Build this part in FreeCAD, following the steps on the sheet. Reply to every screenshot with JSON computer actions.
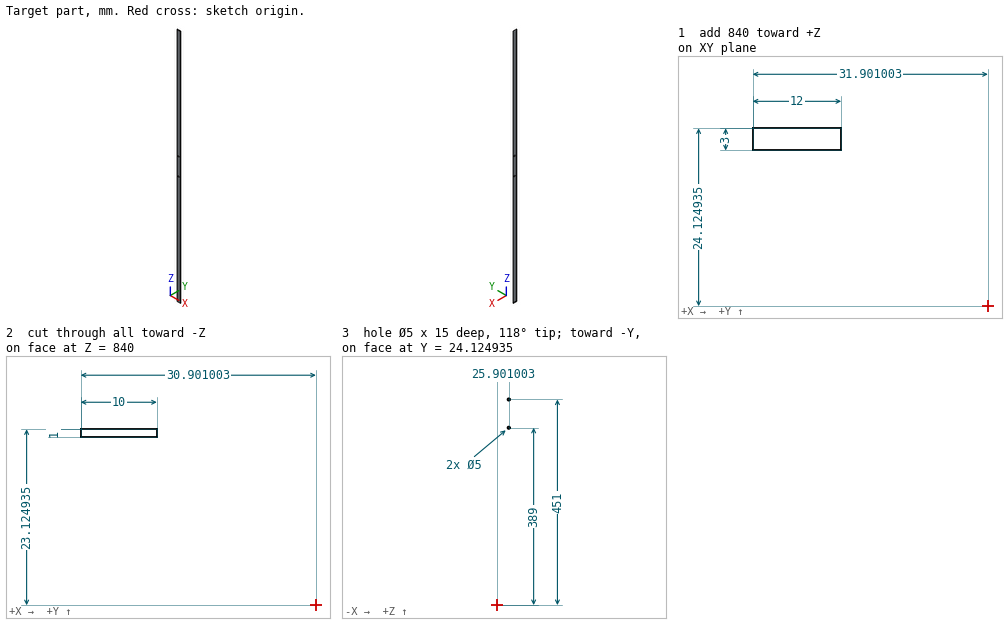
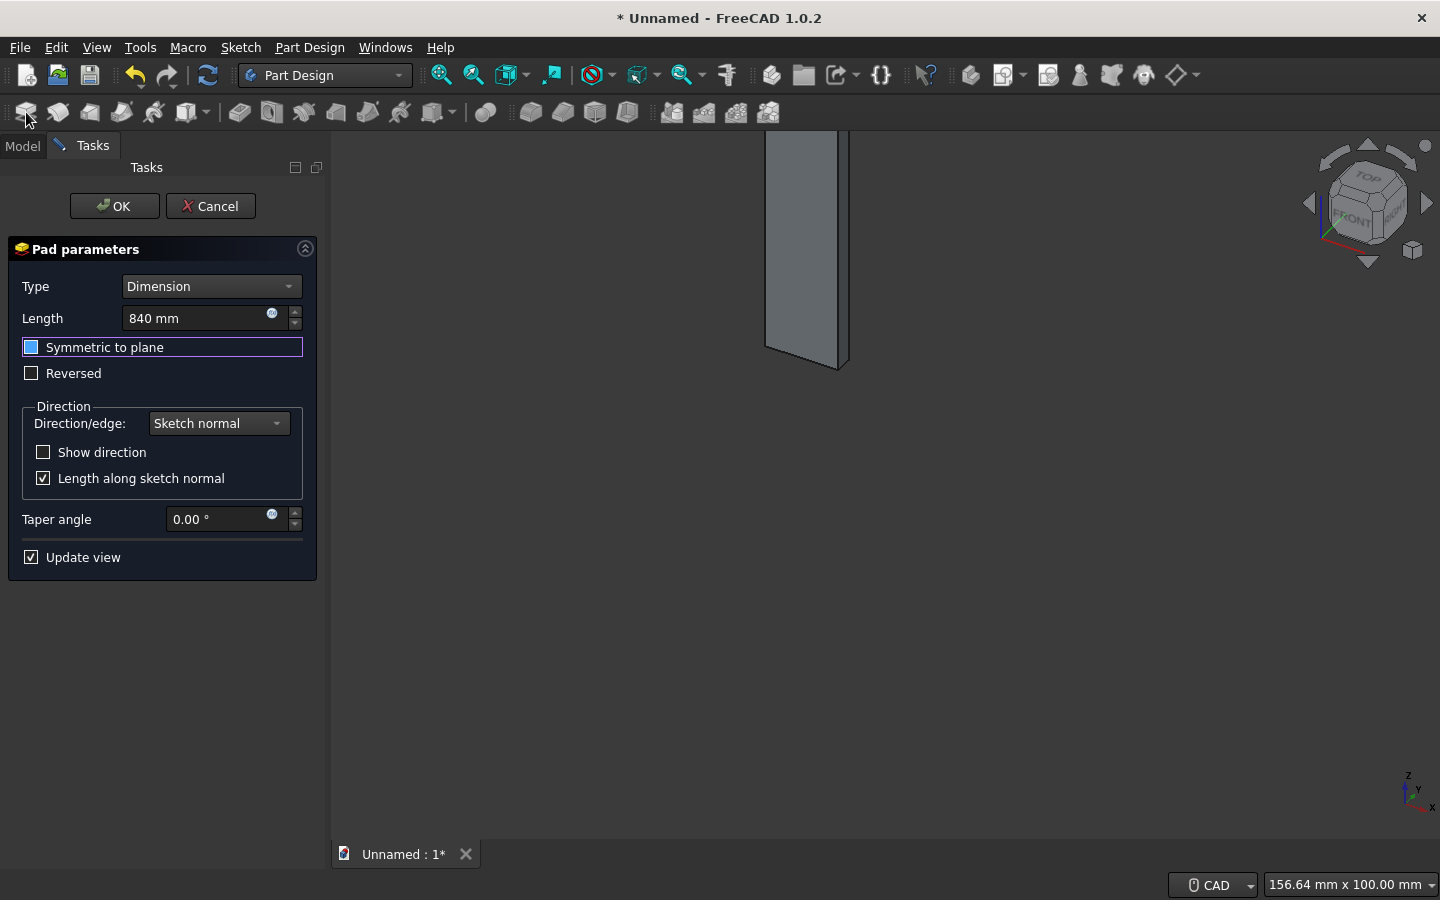
{"action": "left_click", "coordinate": [115, 206]}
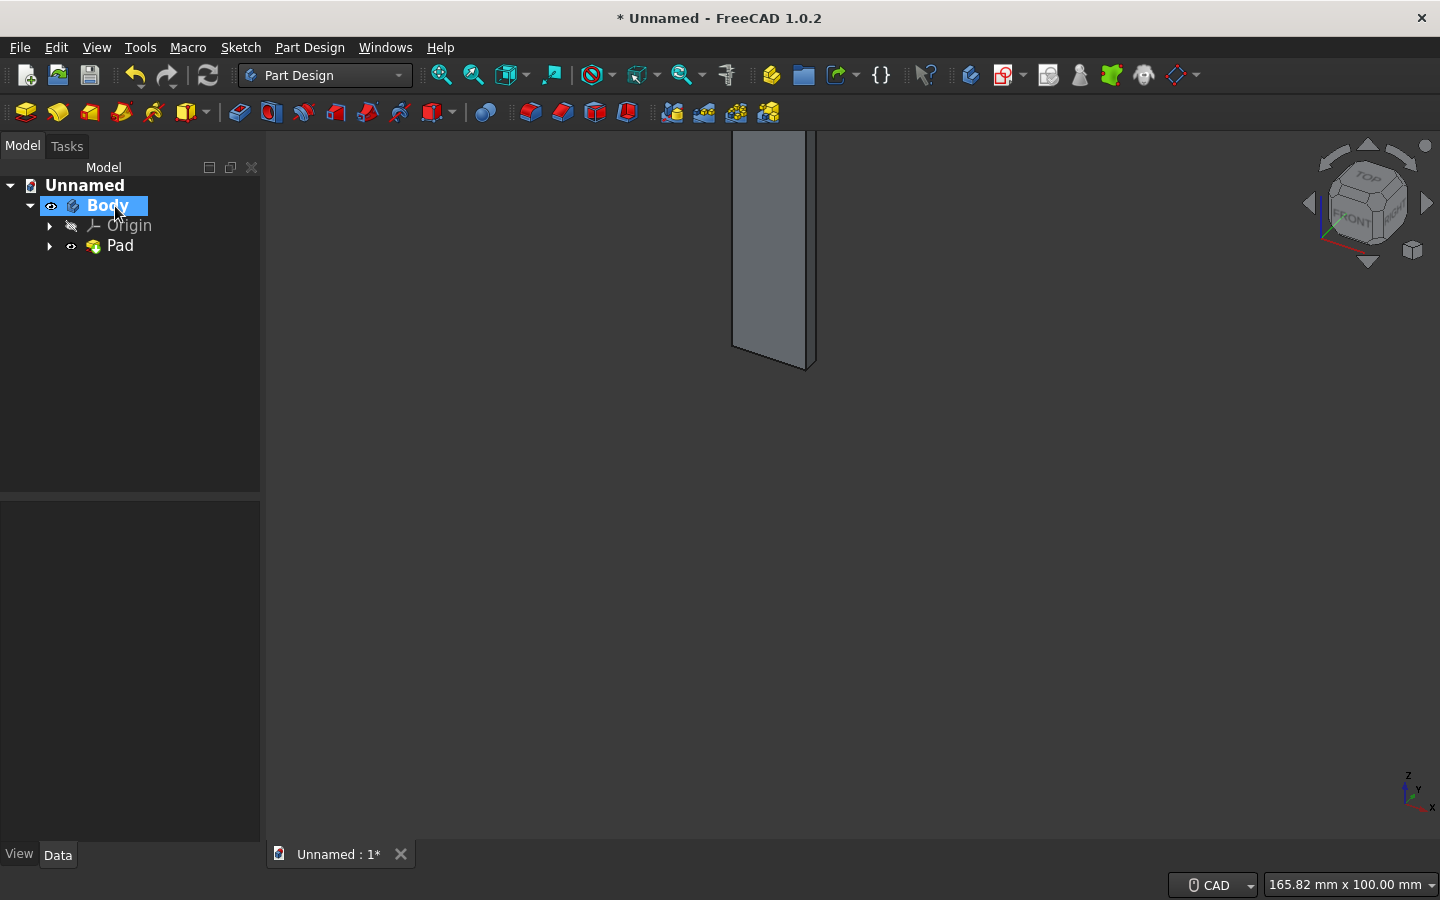
{"action": "left_click", "coordinate": [442, 76]}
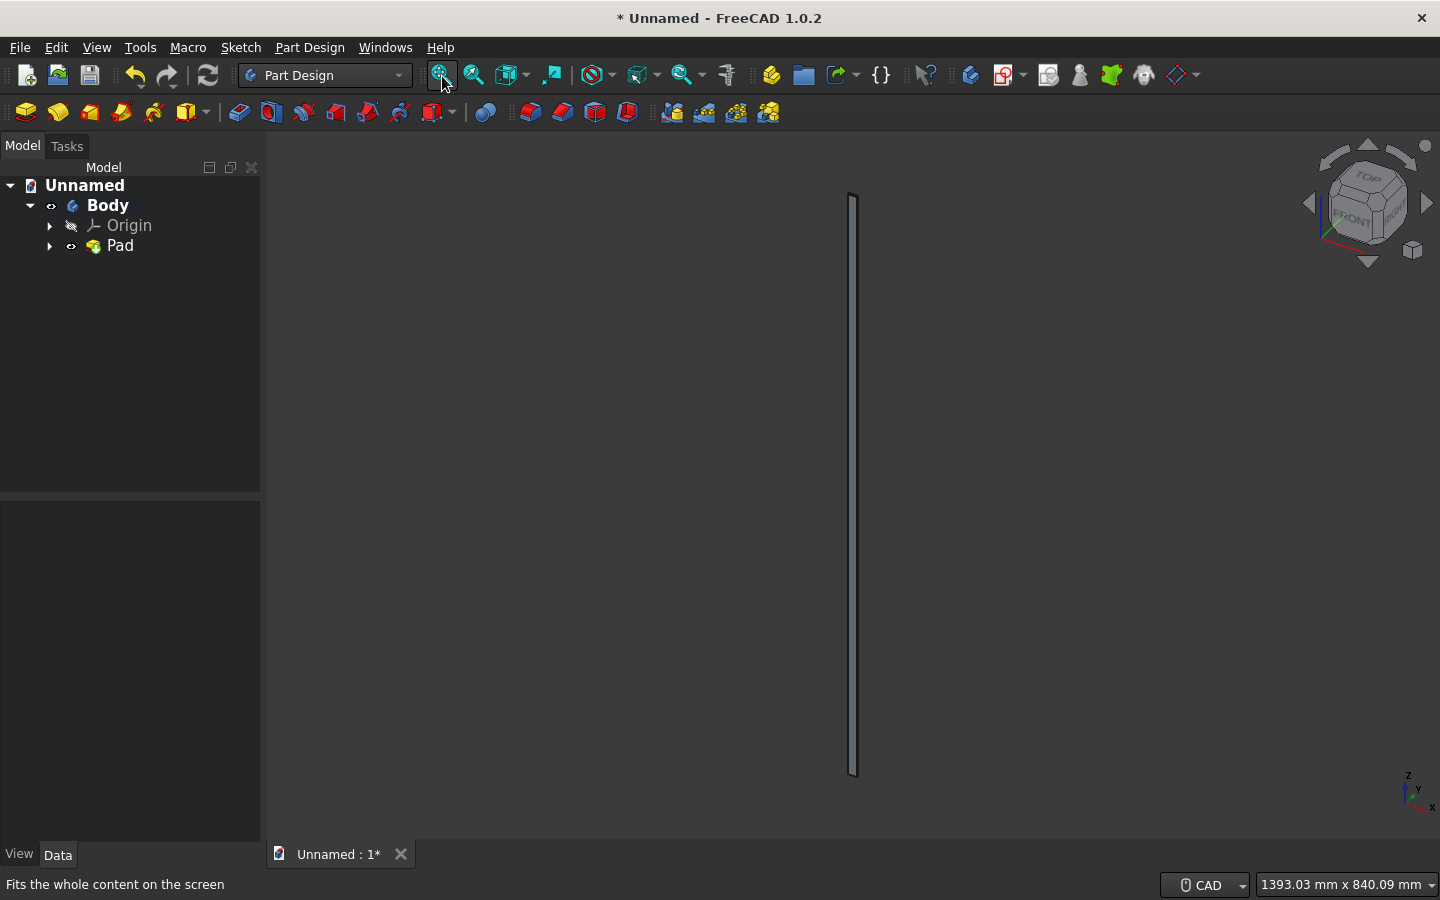
{"action": "scroll", "coordinate": [856, 195], "scroll_direction": "up", "scroll_amount": 12}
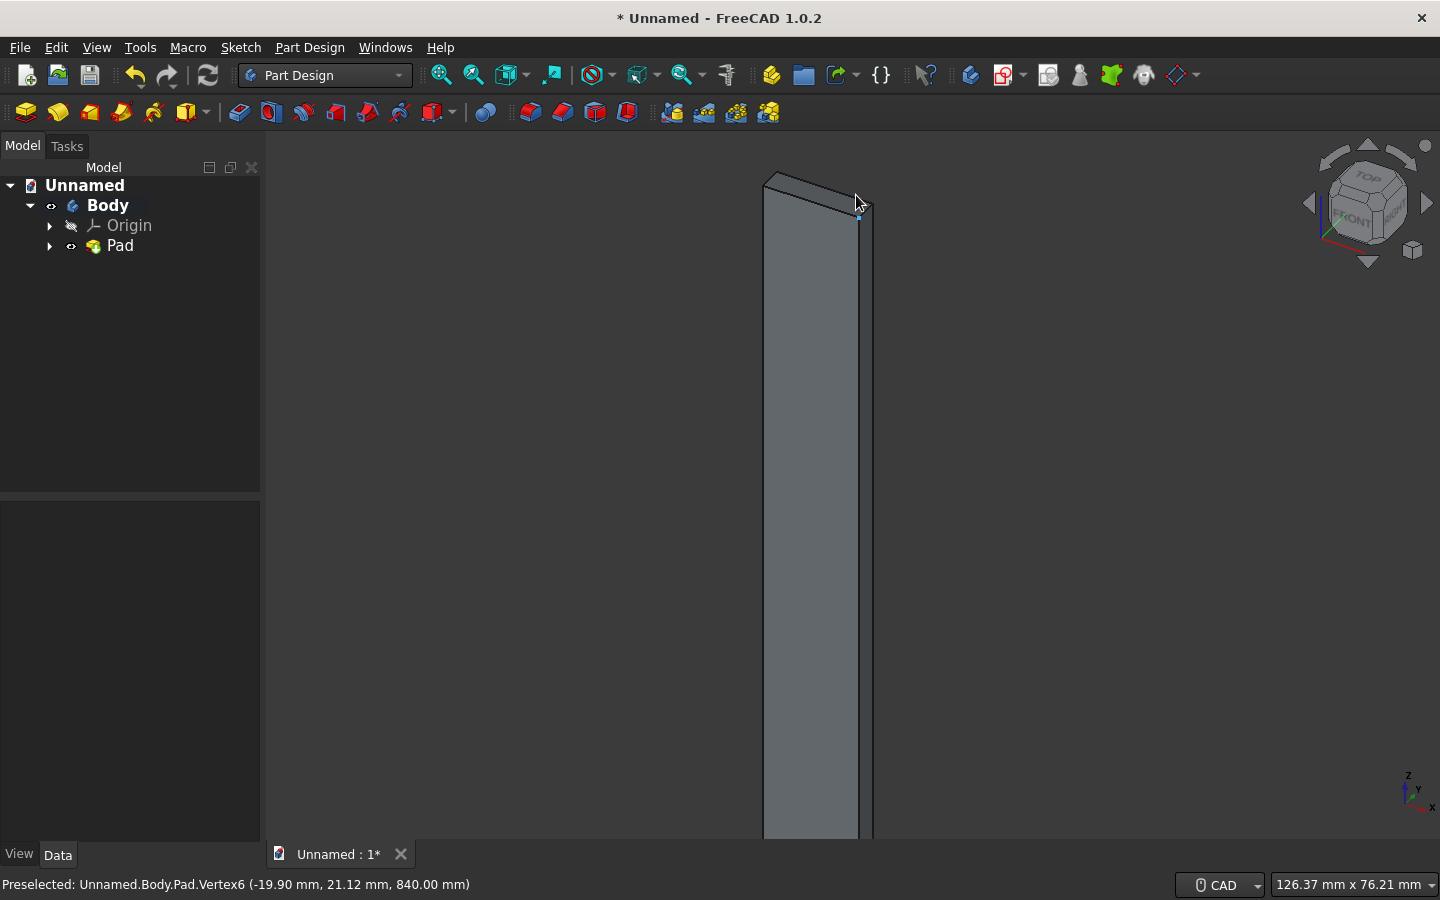
{"action": "left_click", "coordinate": [832, 198]}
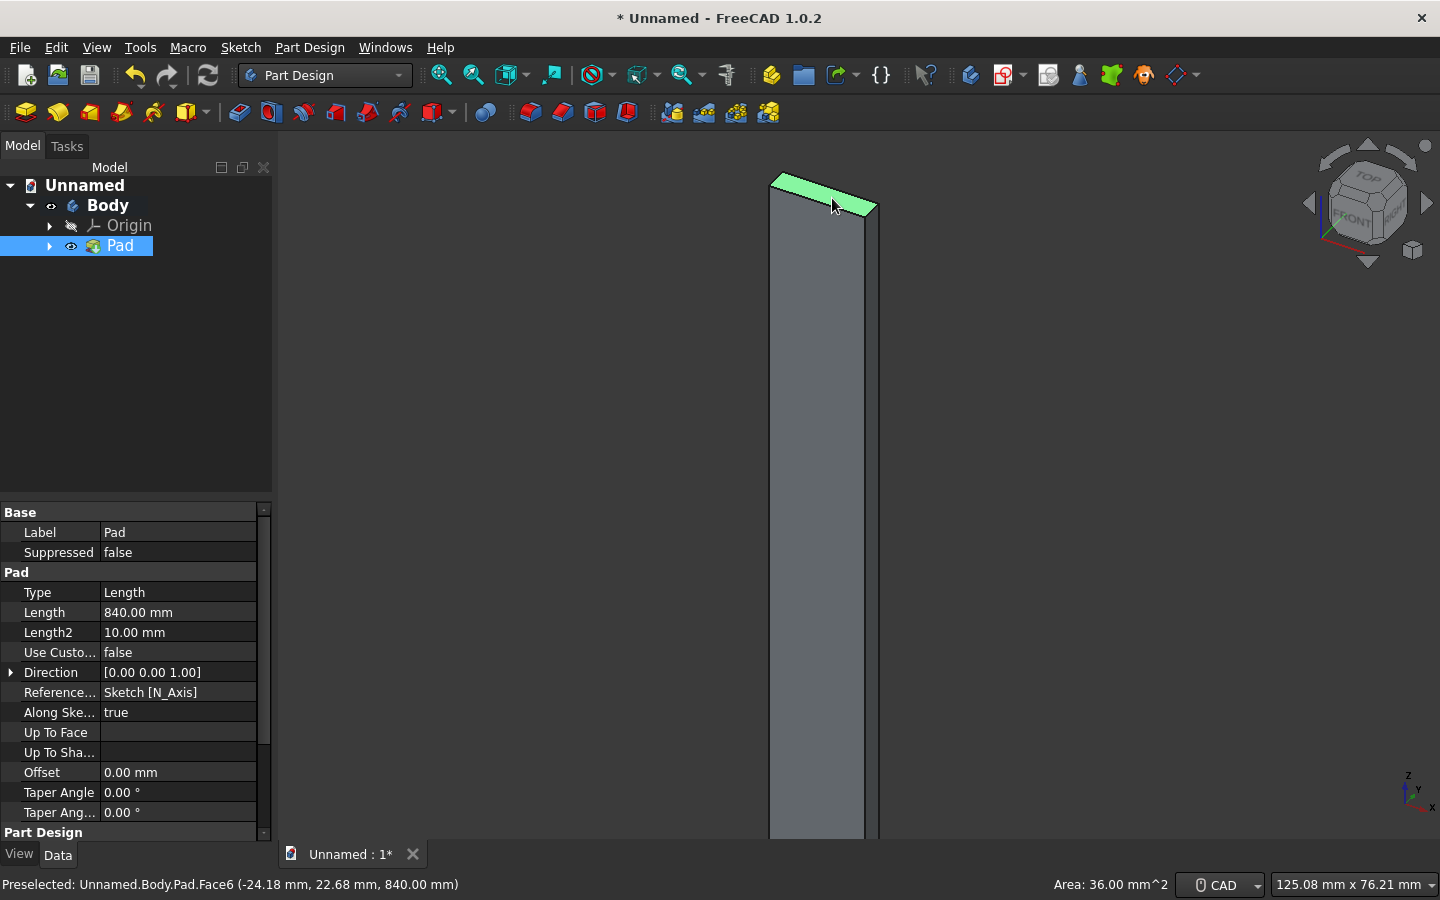
{"action": "left_click", "coordinate": [1004, 76]}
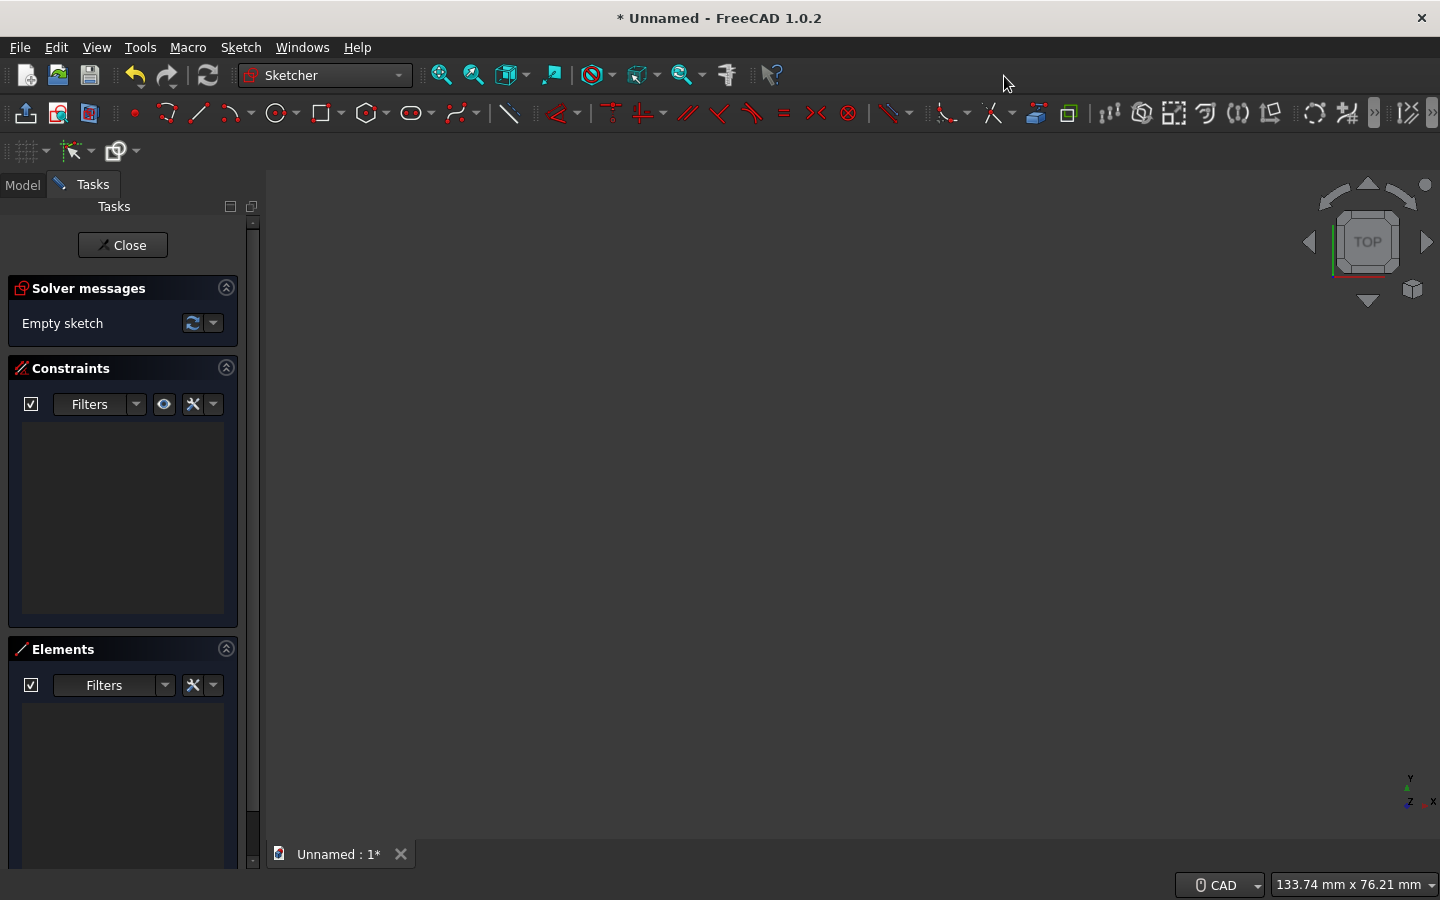
{"action": "scroll", "coordinate": [784, 504], "scroll_direction": "down", "scroll_amount": 5}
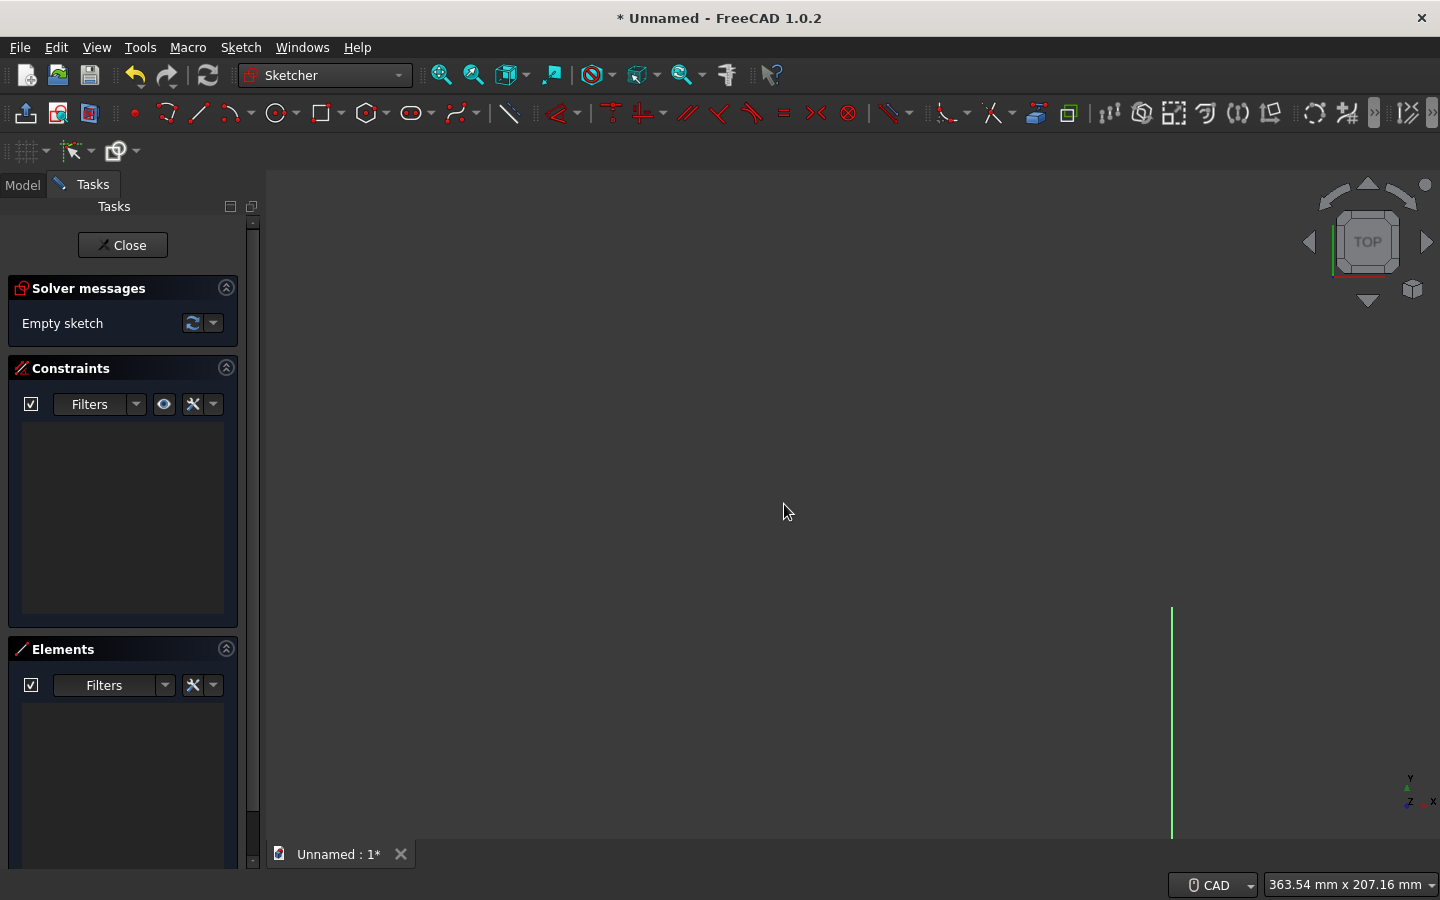
{"action": "scroll", "coordinate": [784, 504], "scroll_direction": "down", "scroll_amount": 5}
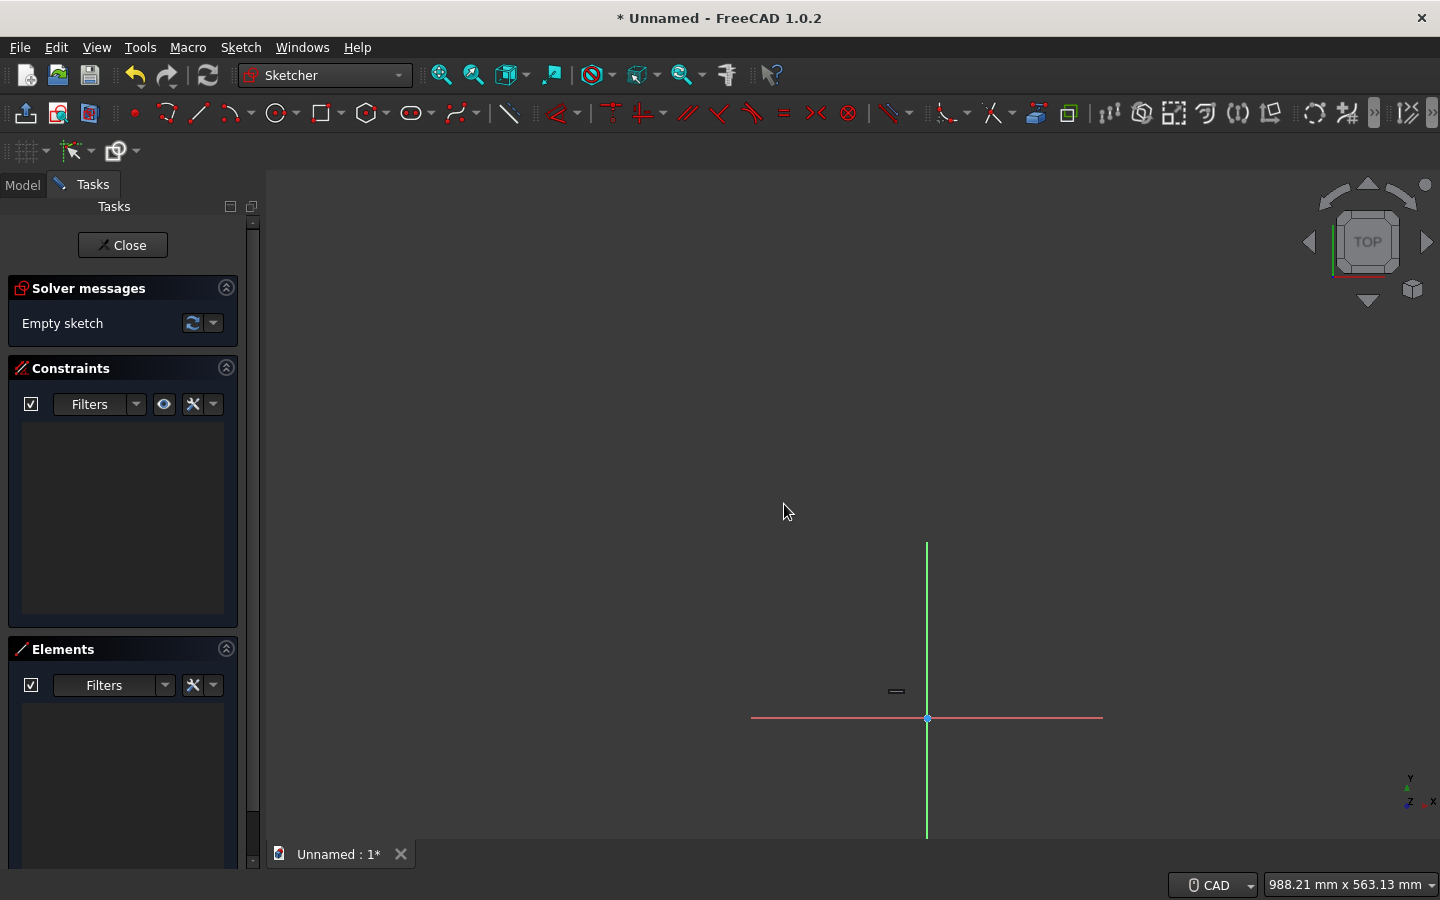
{"action": "scroll", "coordinate": [902, 701], "scroll_direction": "up", "scroll_amount": 15}